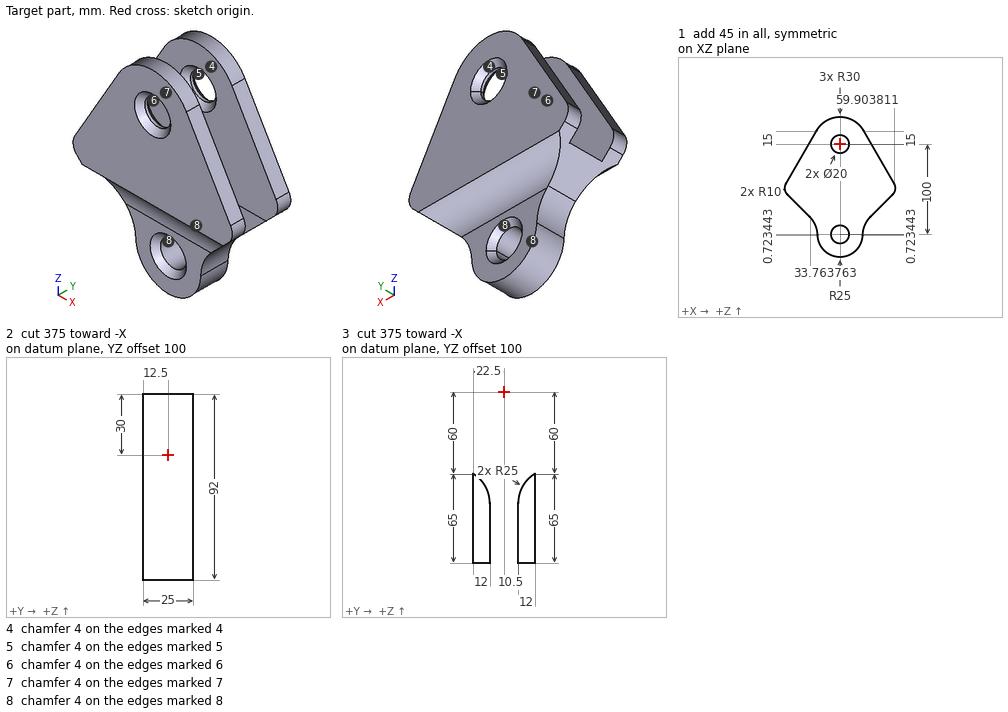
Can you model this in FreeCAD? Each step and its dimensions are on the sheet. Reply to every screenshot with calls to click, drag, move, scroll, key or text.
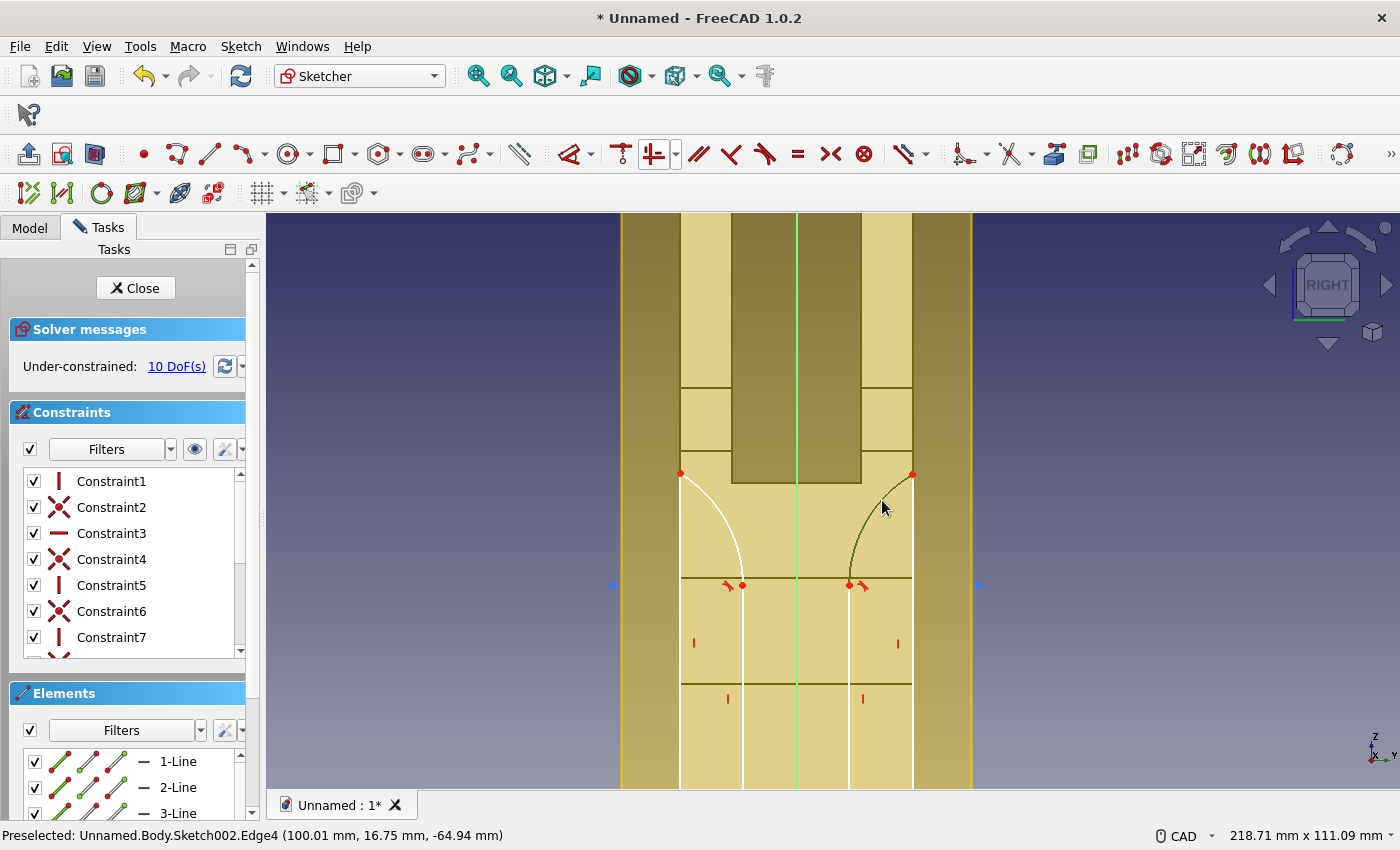
click(737, 546)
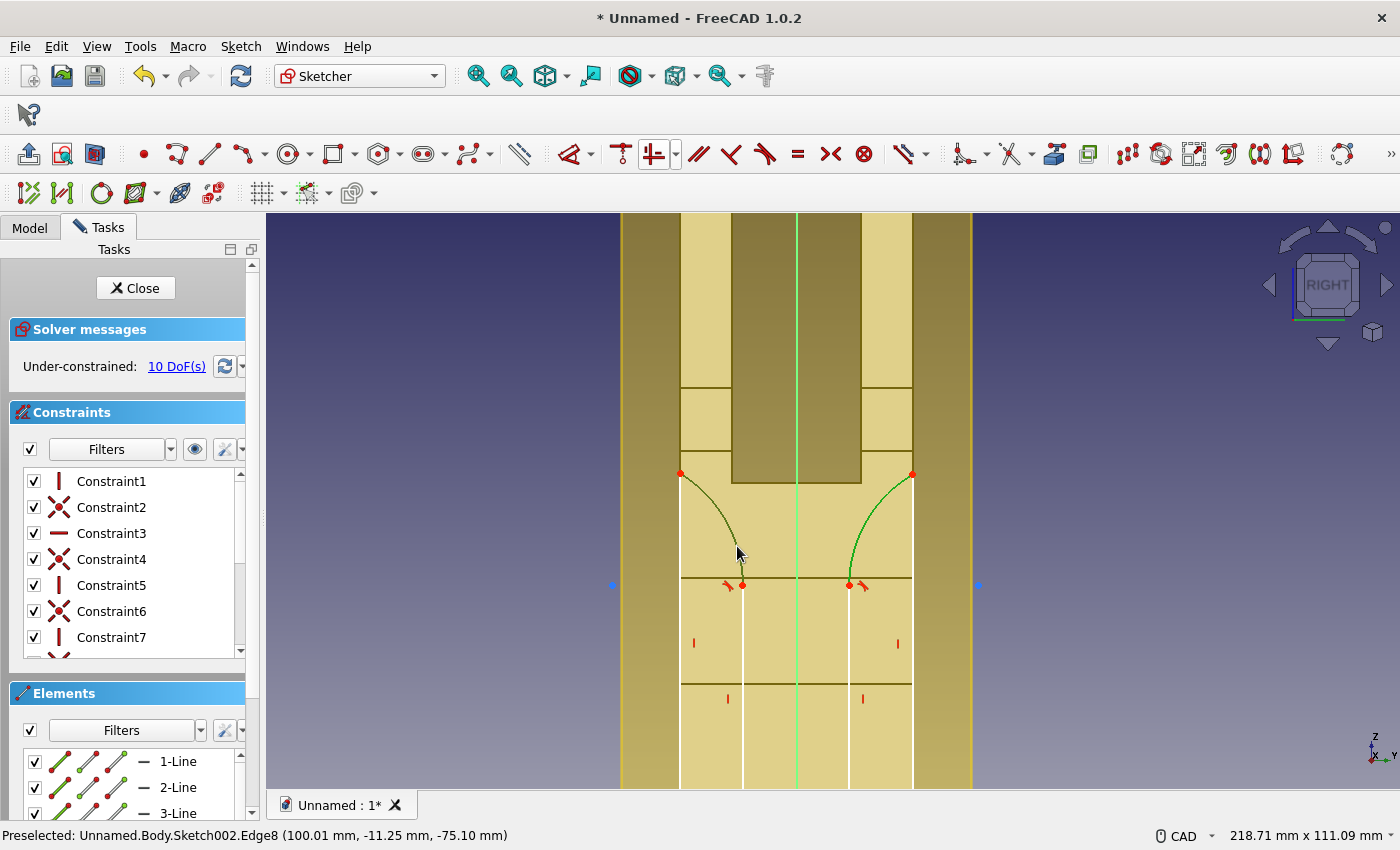
click(798, 154)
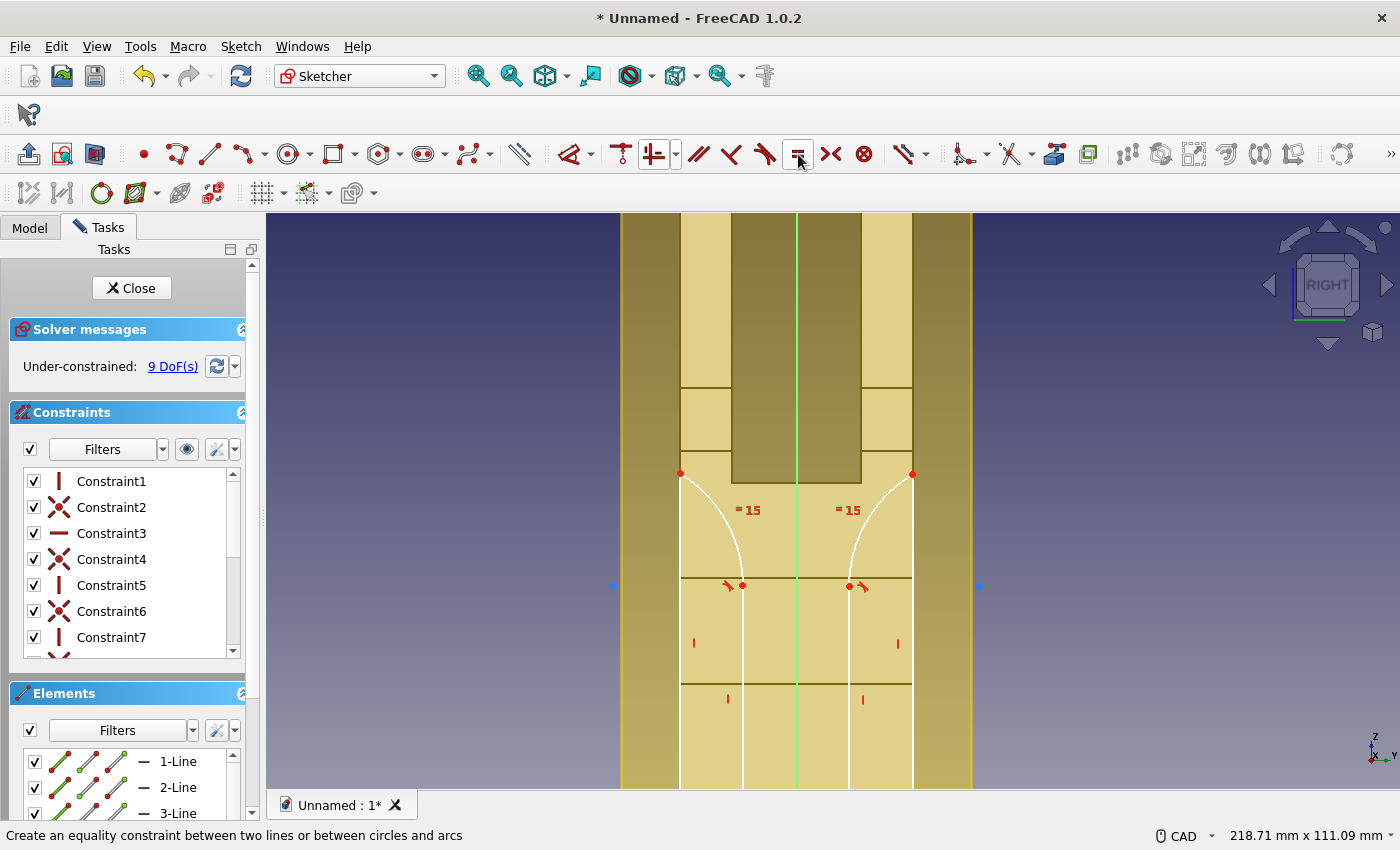
click(568, 154)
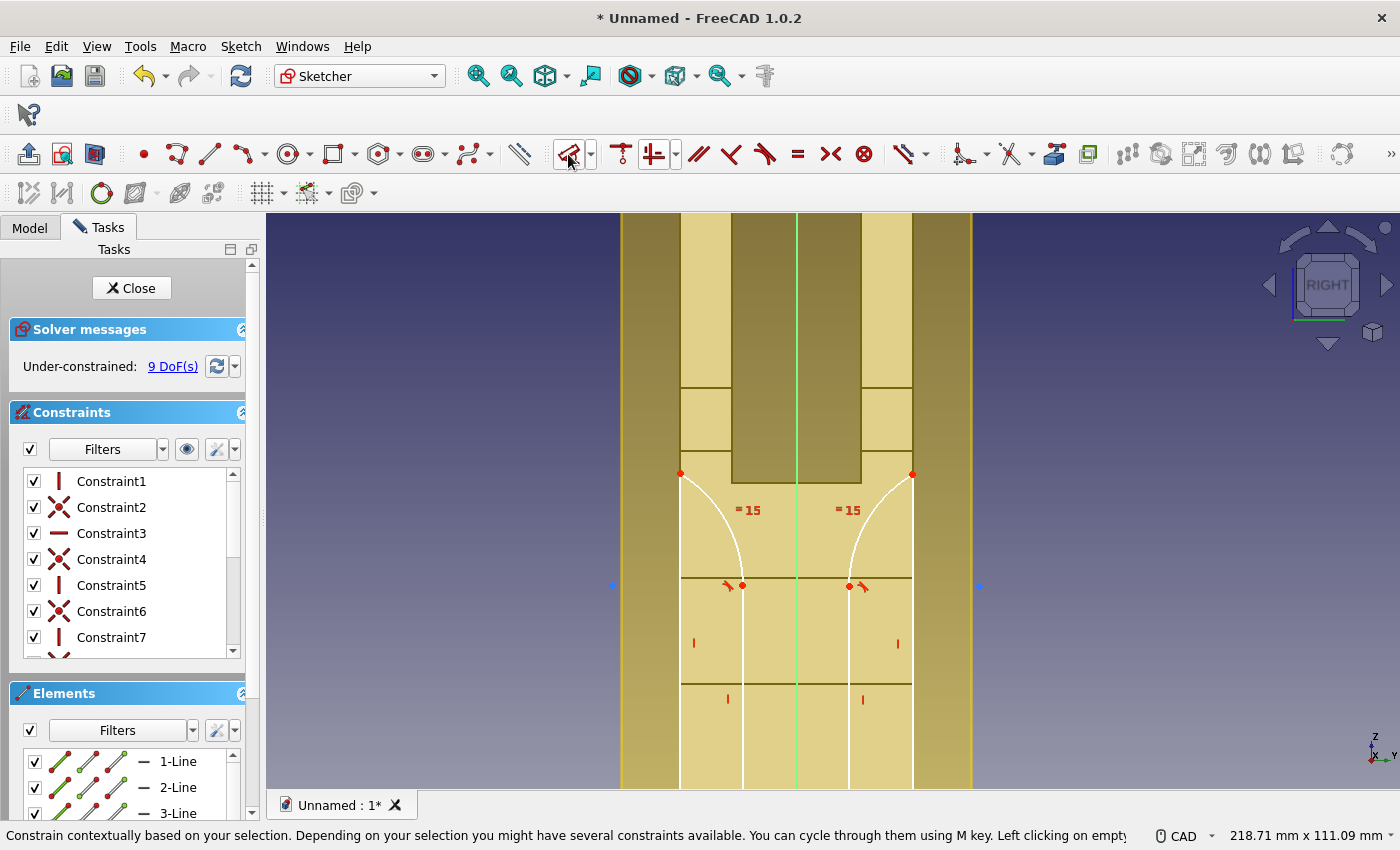
click(882, 500)
click(858, 479)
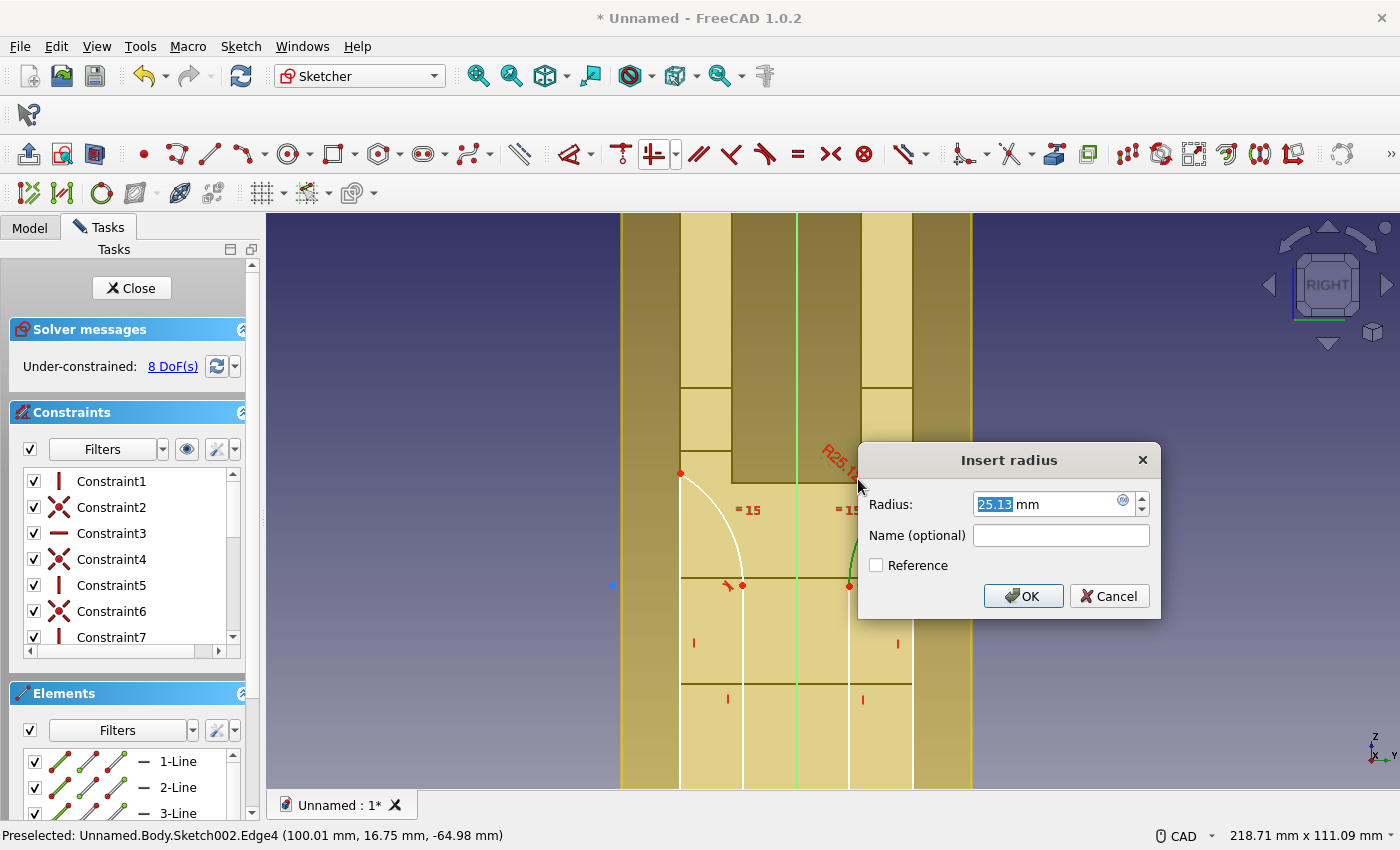
text(25)
key(Return)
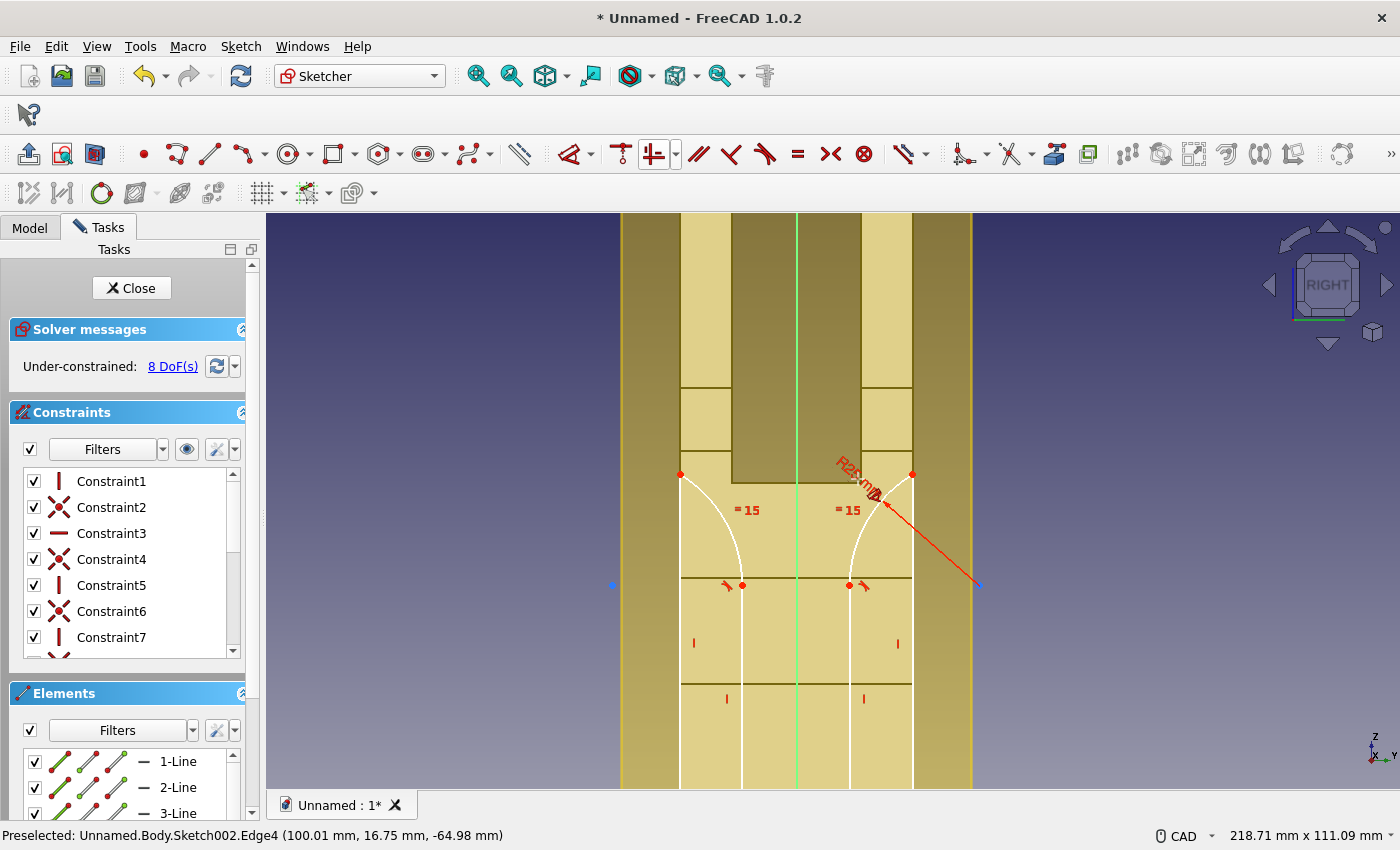
scroll(725, 520, down, 3)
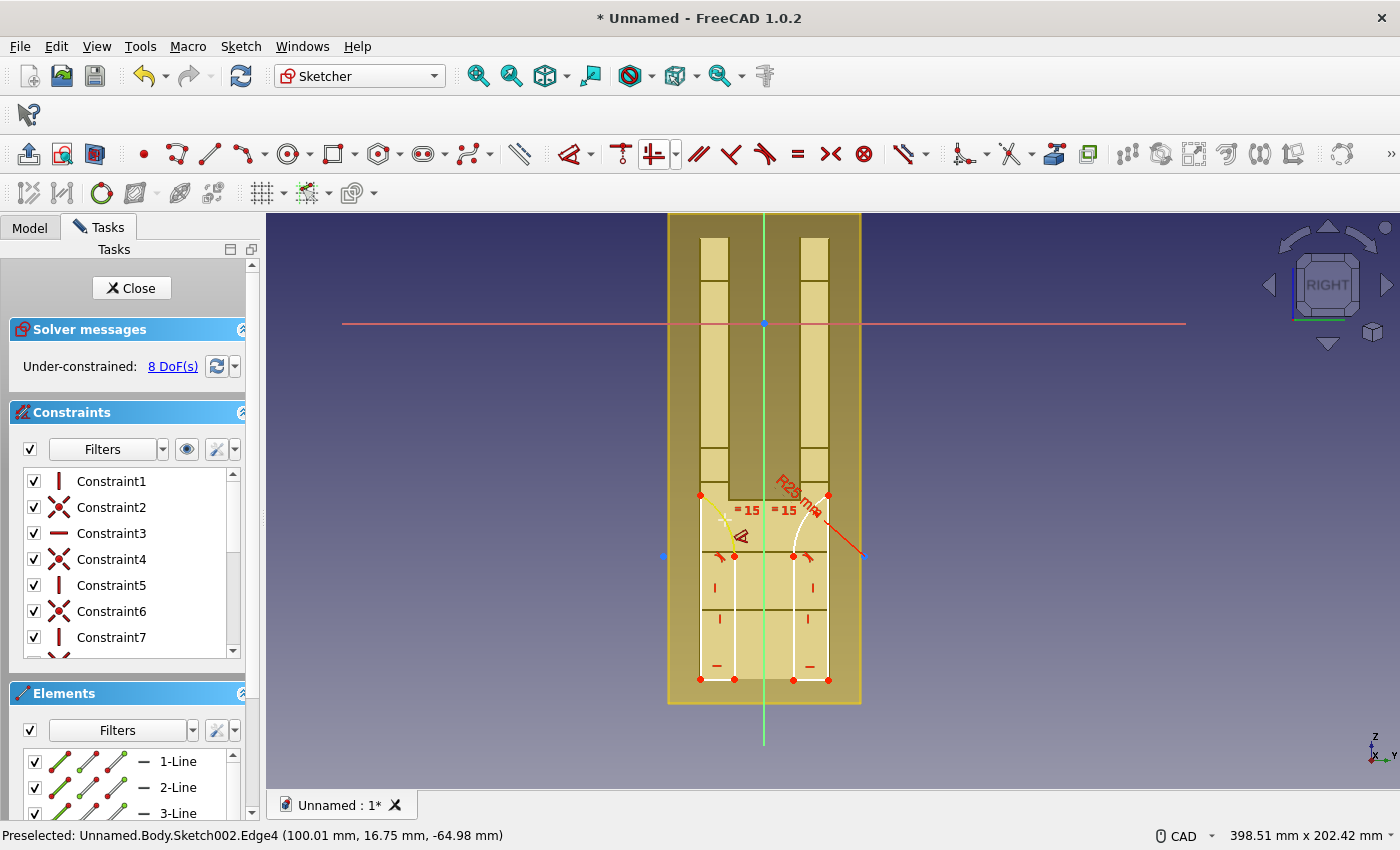
scroll(804, 680, up, 2)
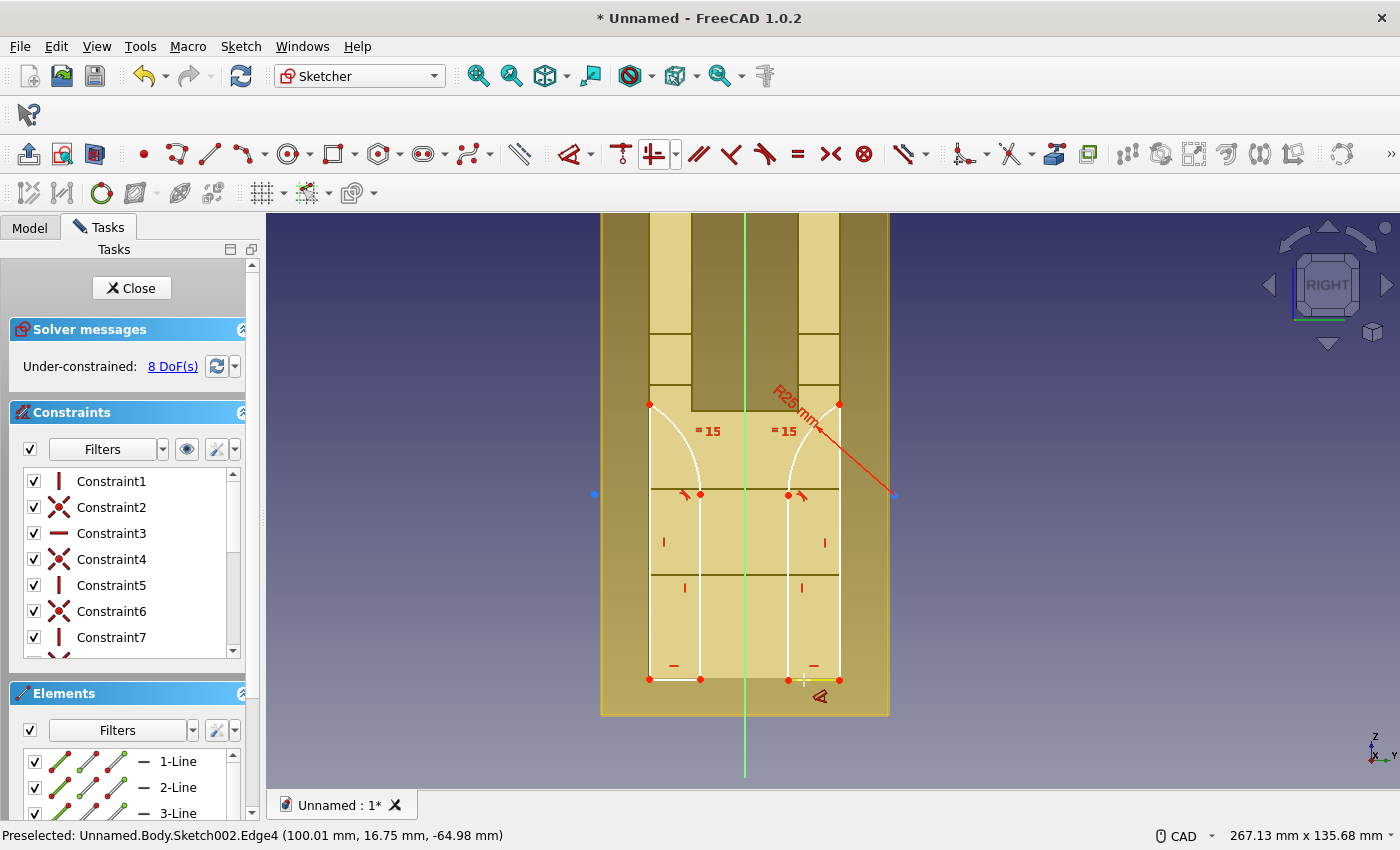
click(804, 680)
click(814, 714)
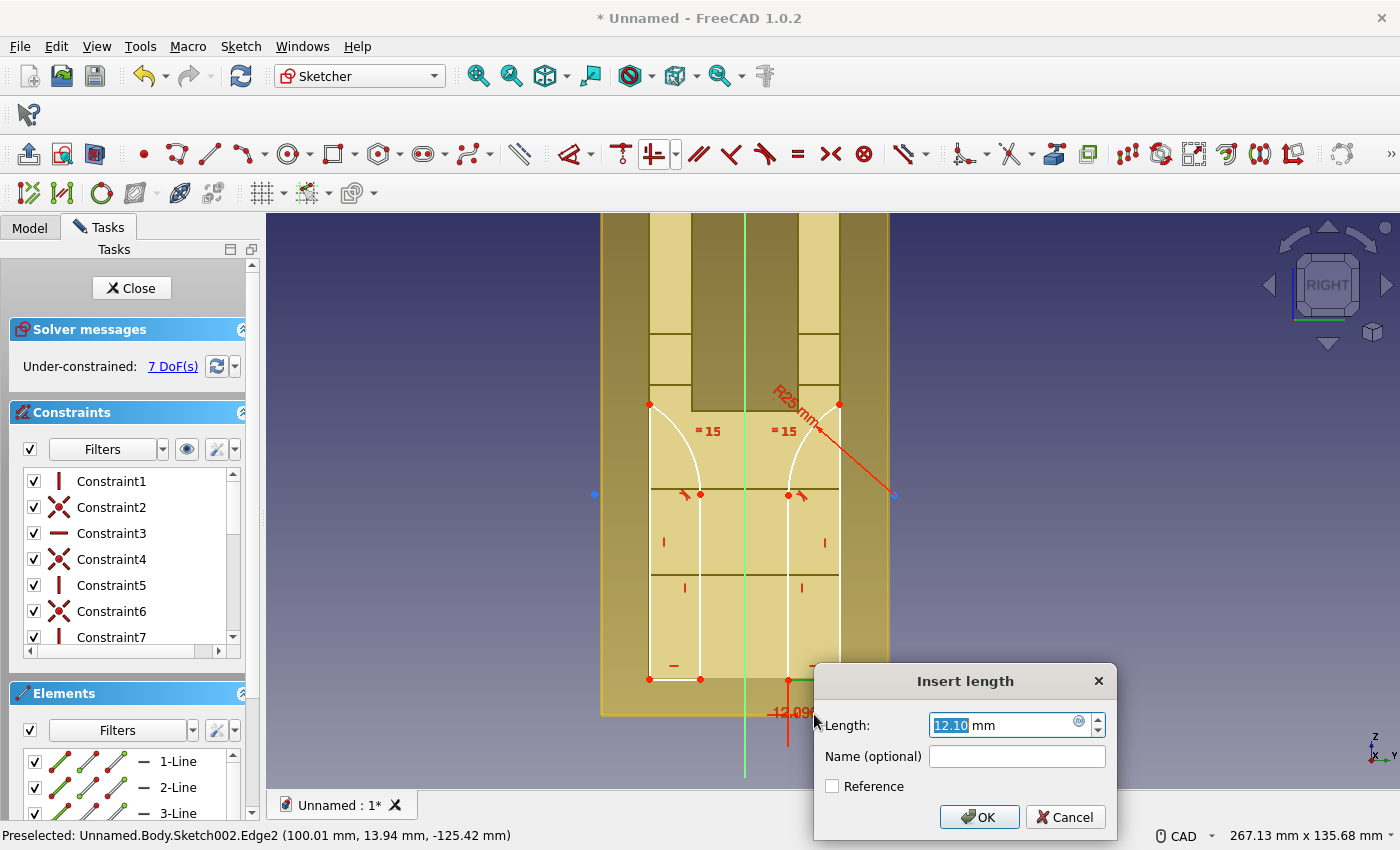
text(12)
key(Return)